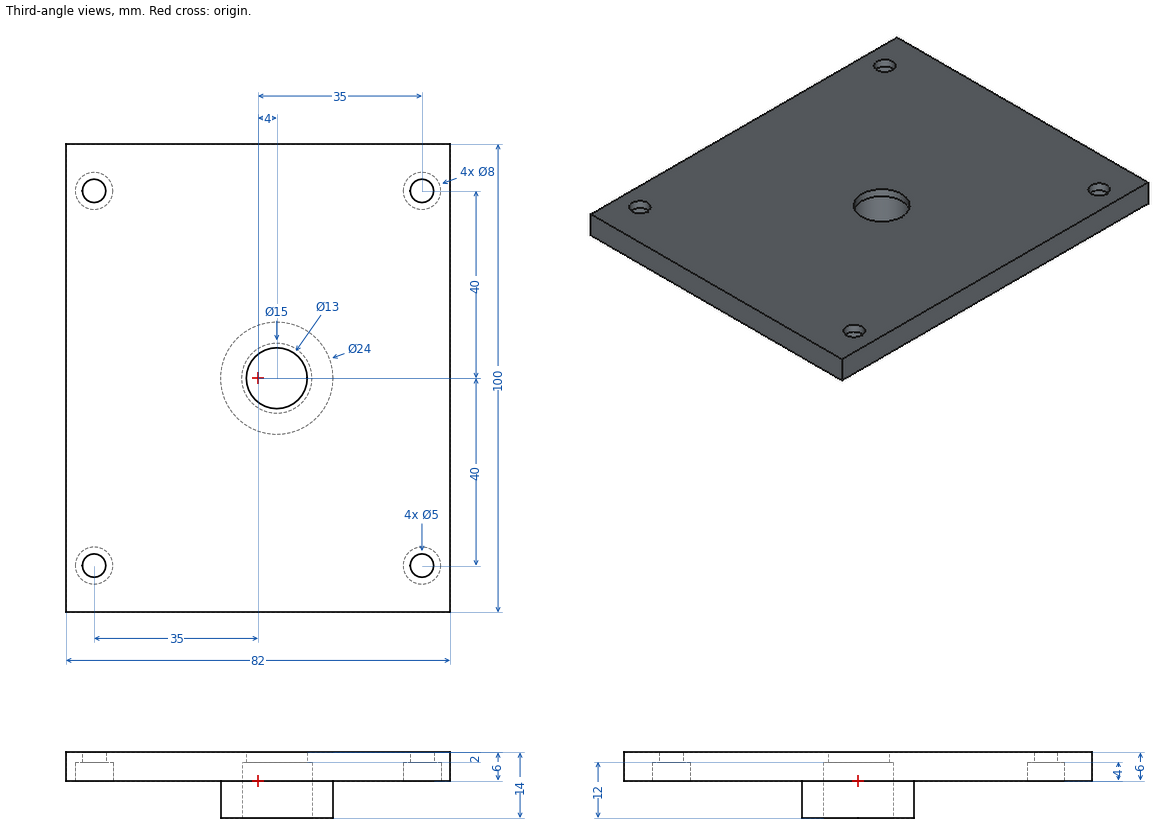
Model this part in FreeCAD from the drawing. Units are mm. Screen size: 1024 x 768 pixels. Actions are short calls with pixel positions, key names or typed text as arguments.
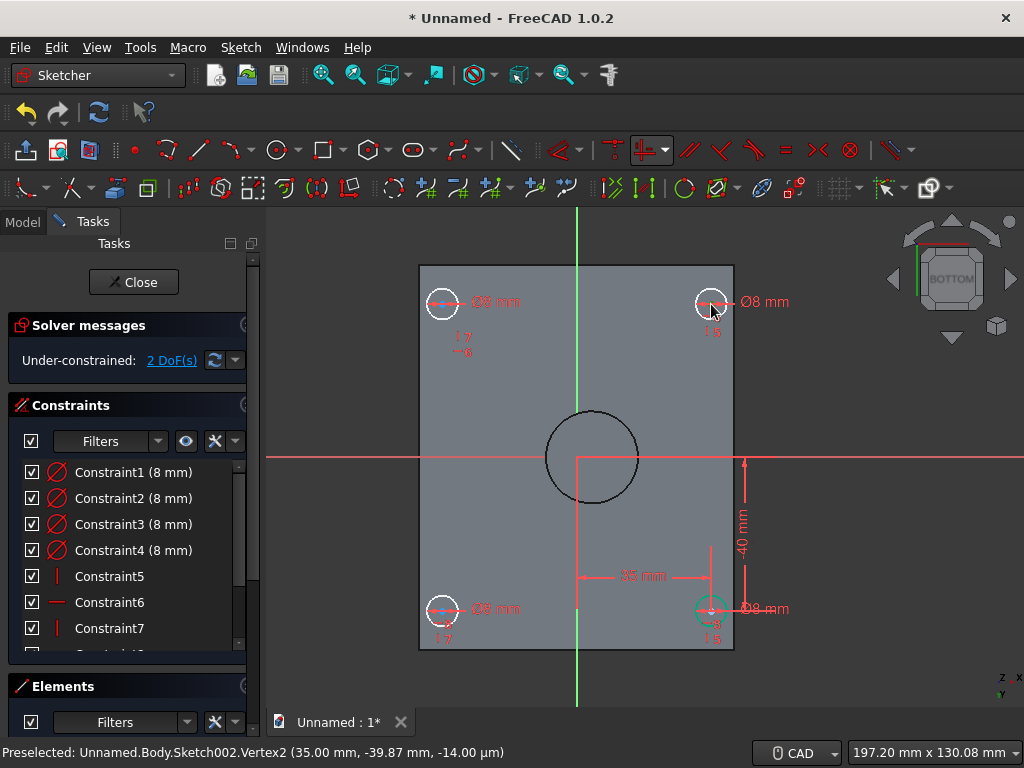
click(582, 150)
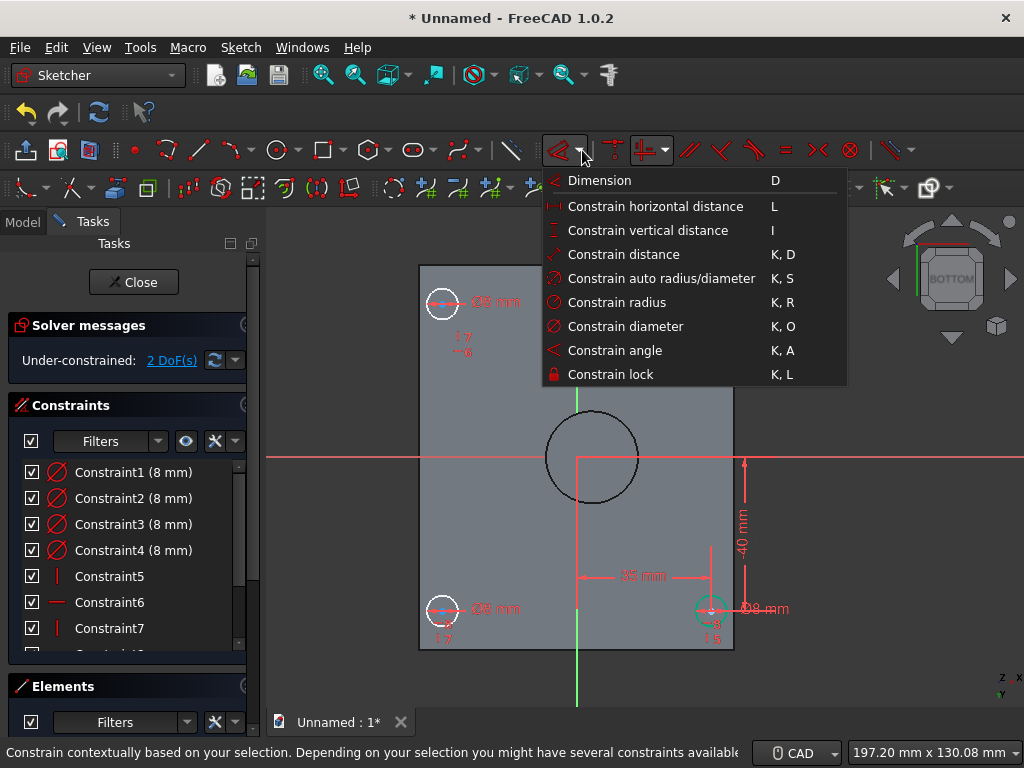
click(695, 230)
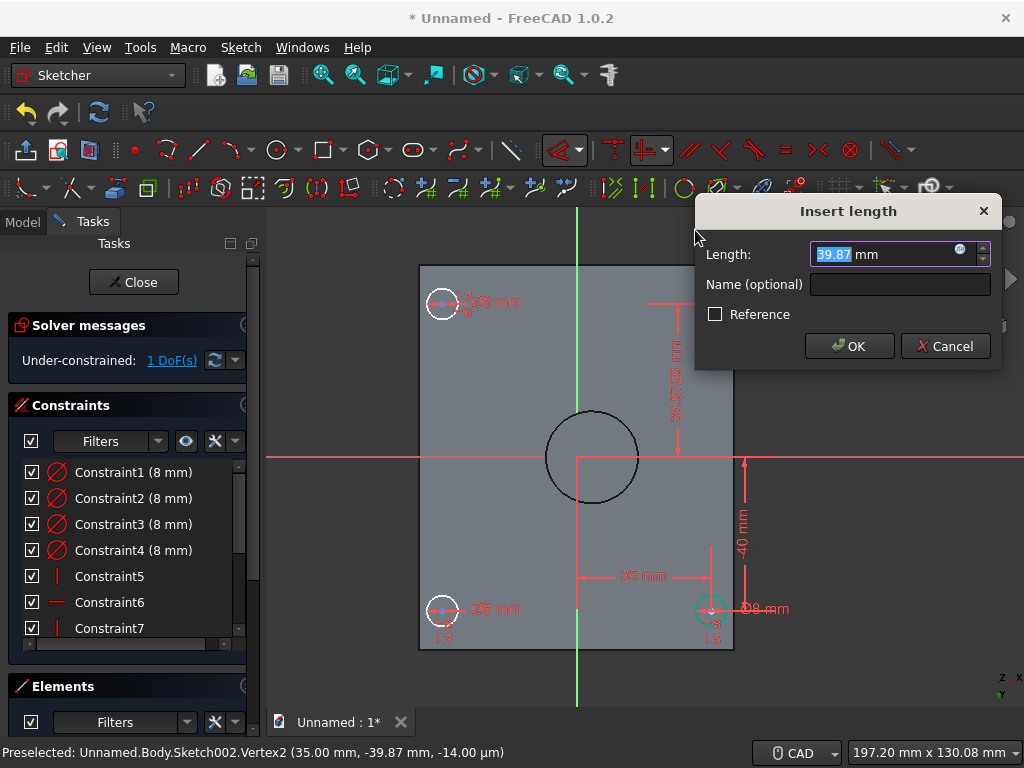
text(40)
key(Return)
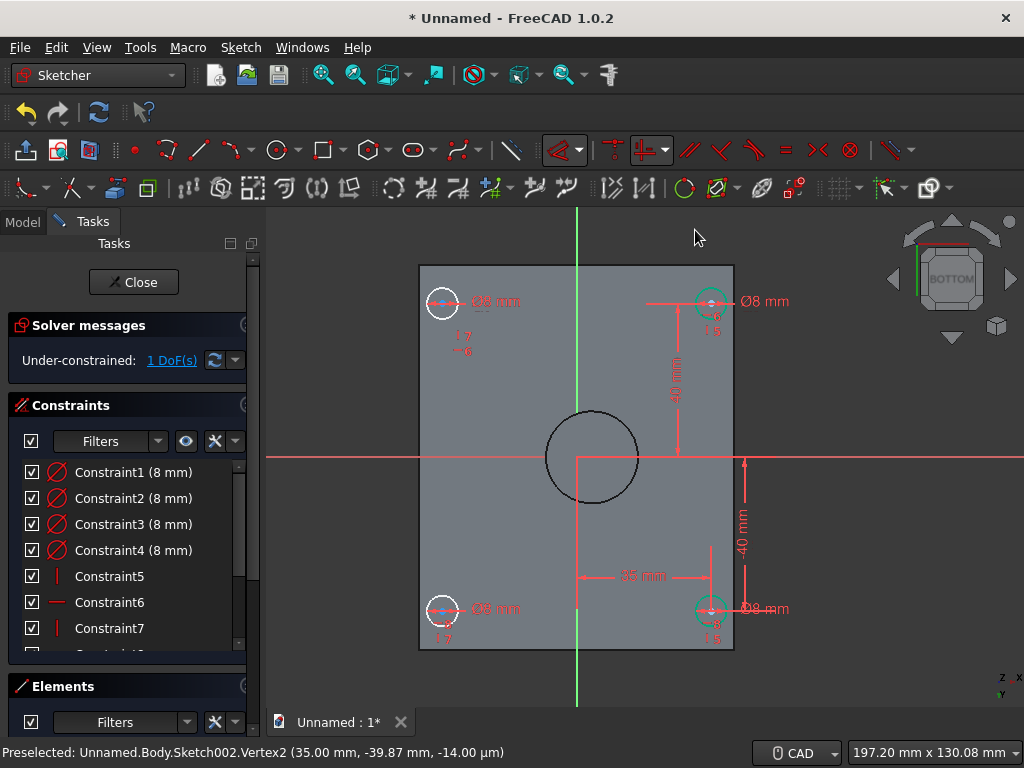
click(442, 304)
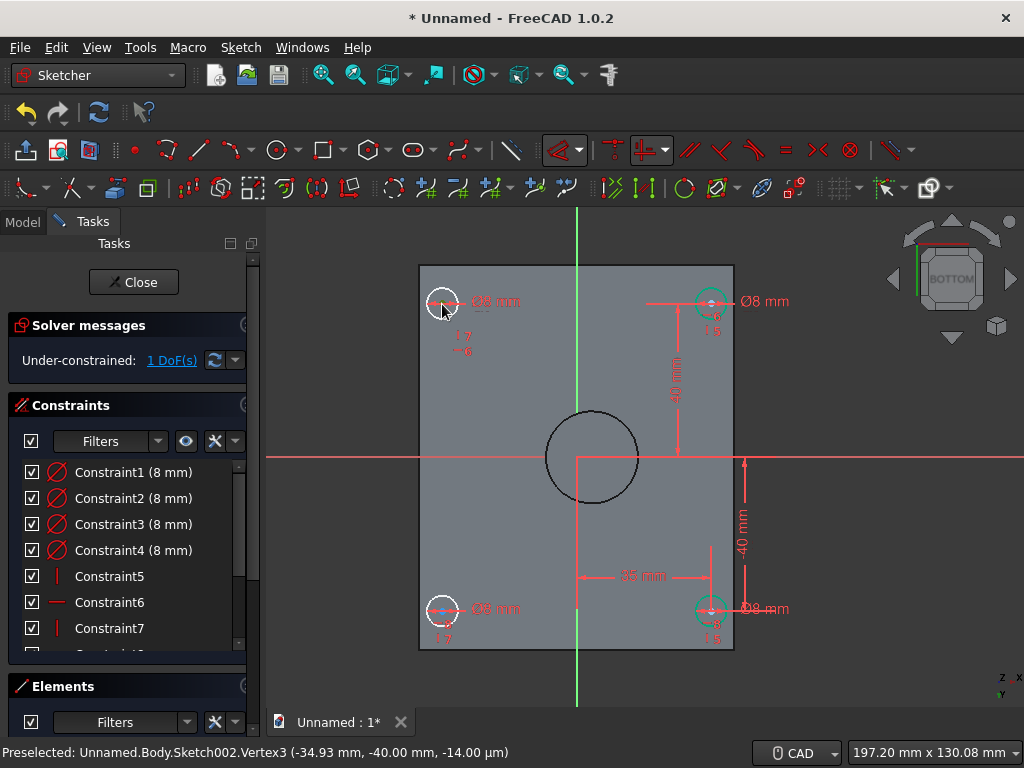
key(l)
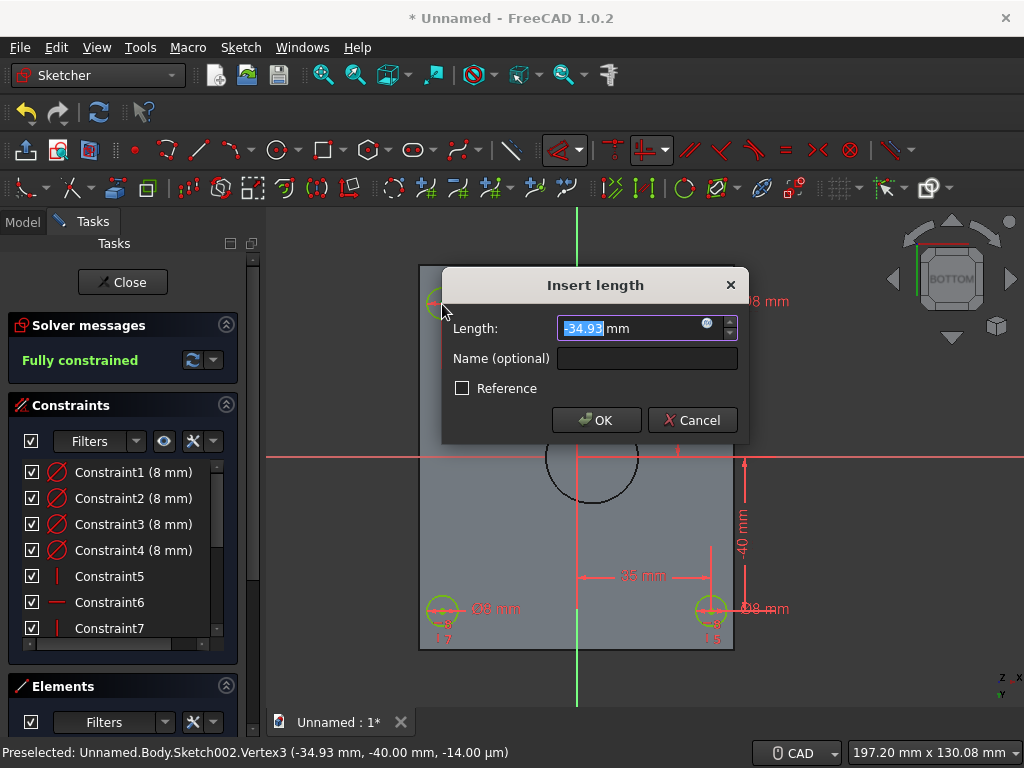
text(-35)
key(Return)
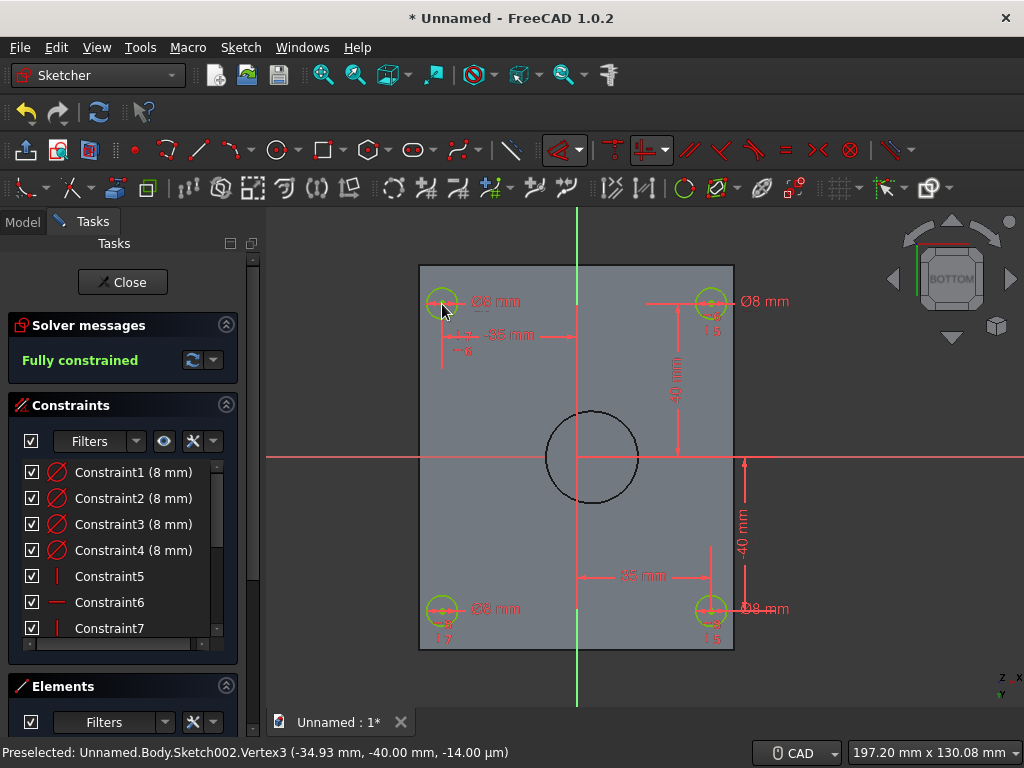
click(123, 282)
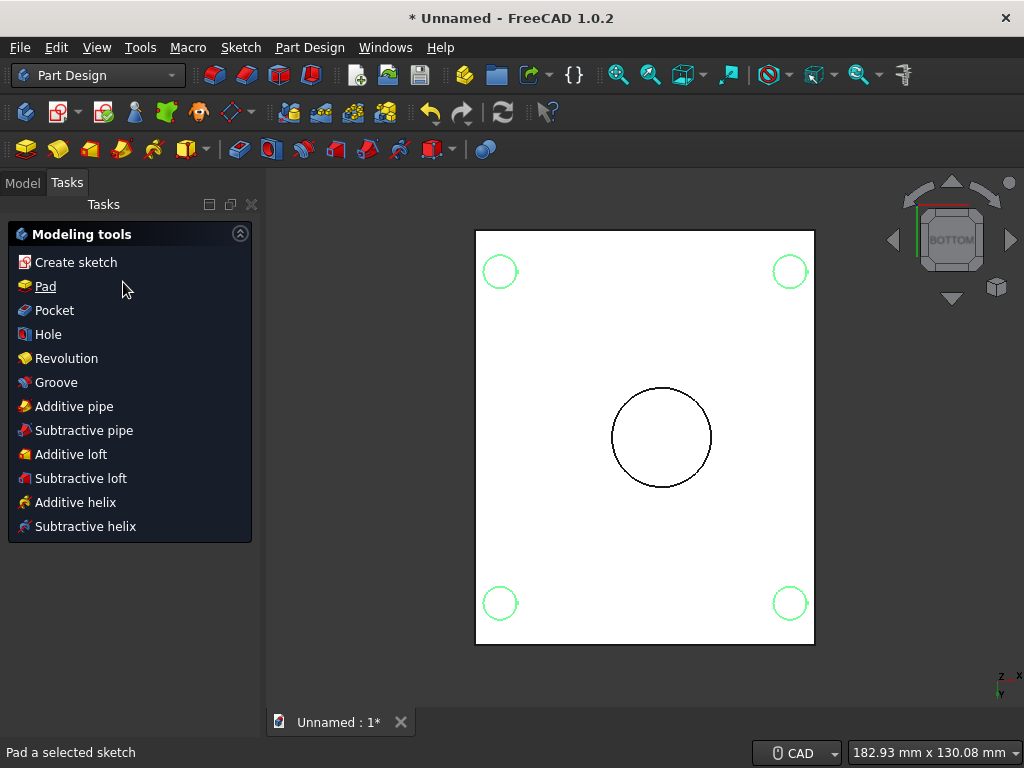
click(240, 150)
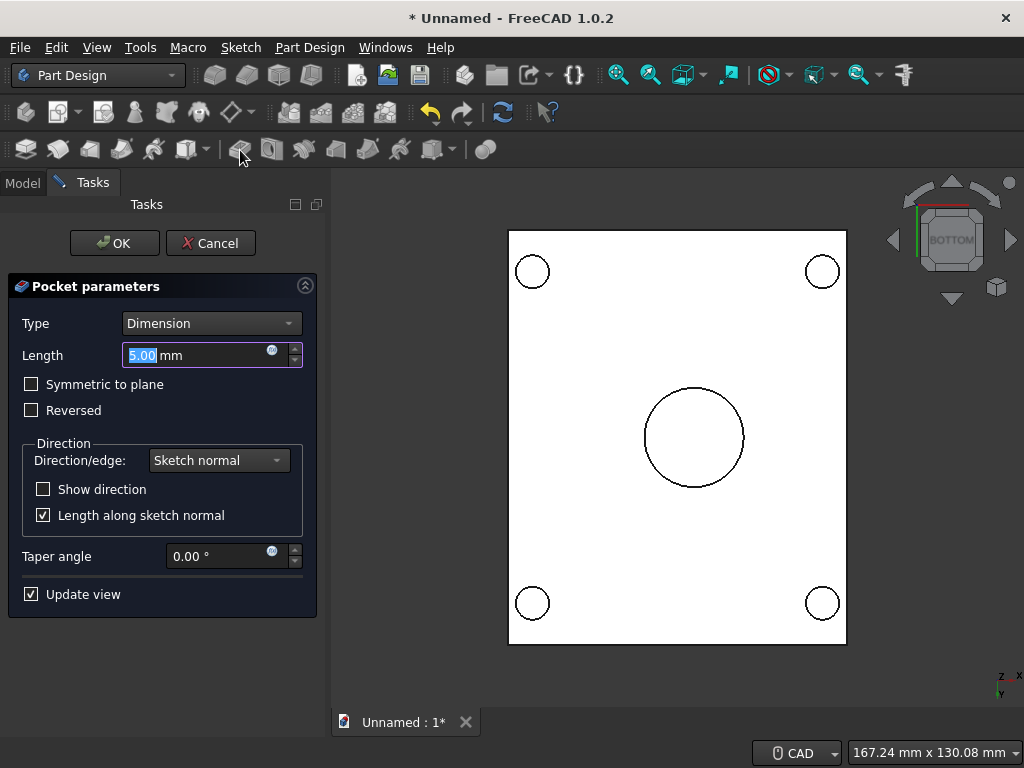
text(4)
key(Tab)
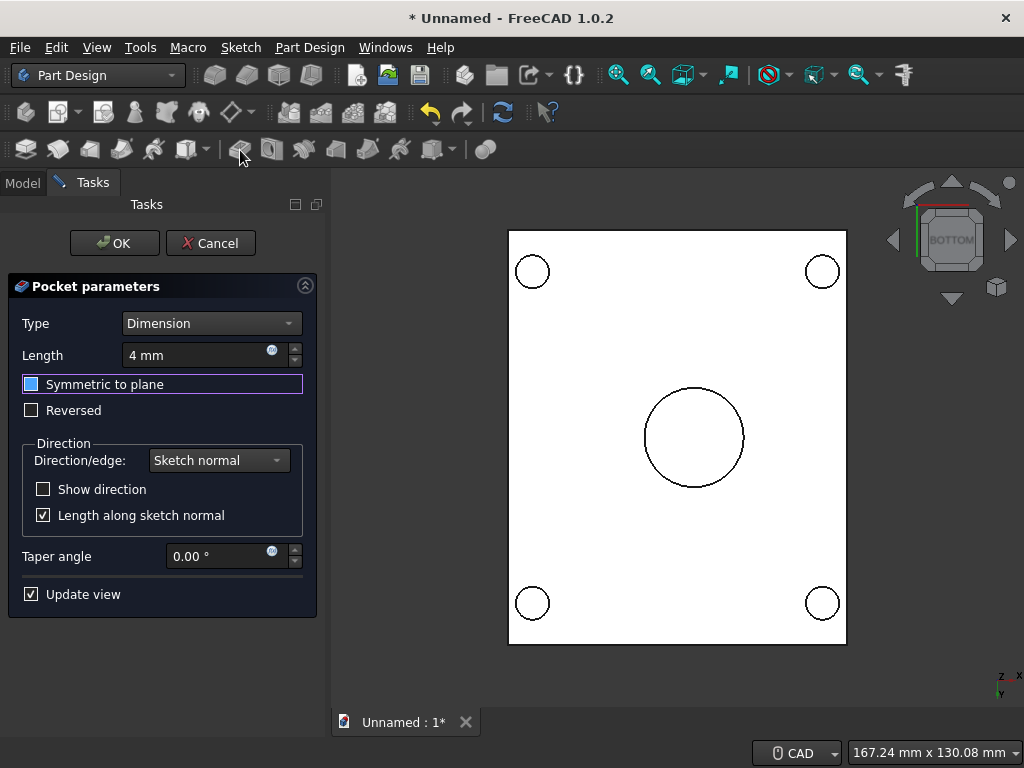
click(115, 243)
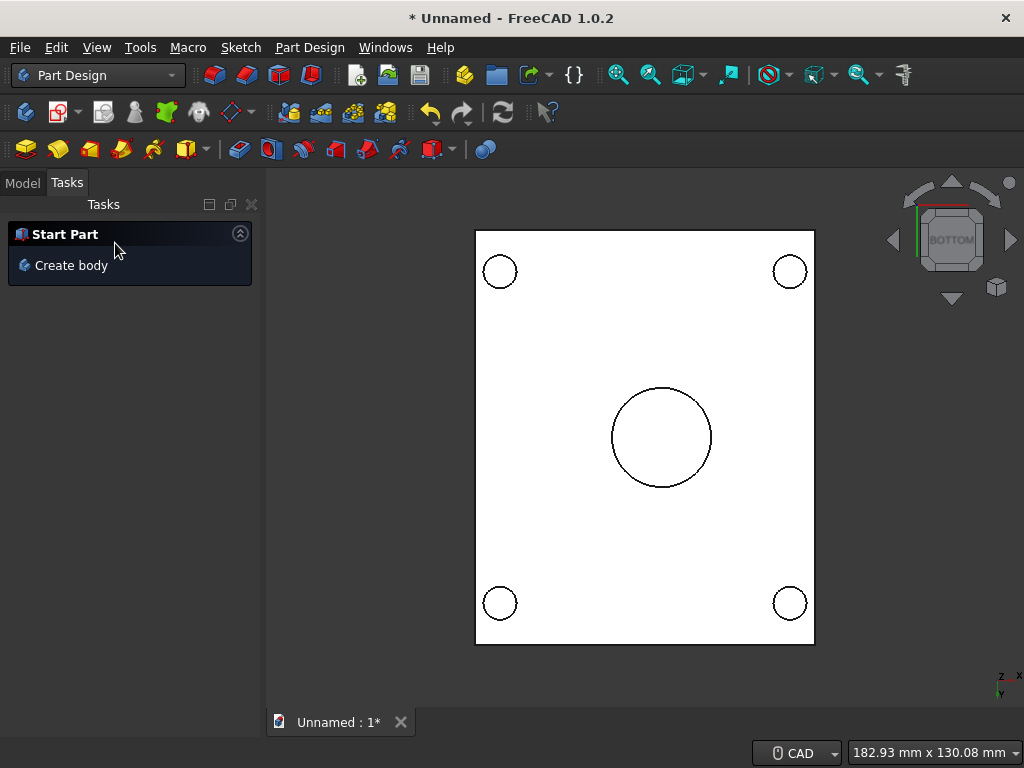
key(0)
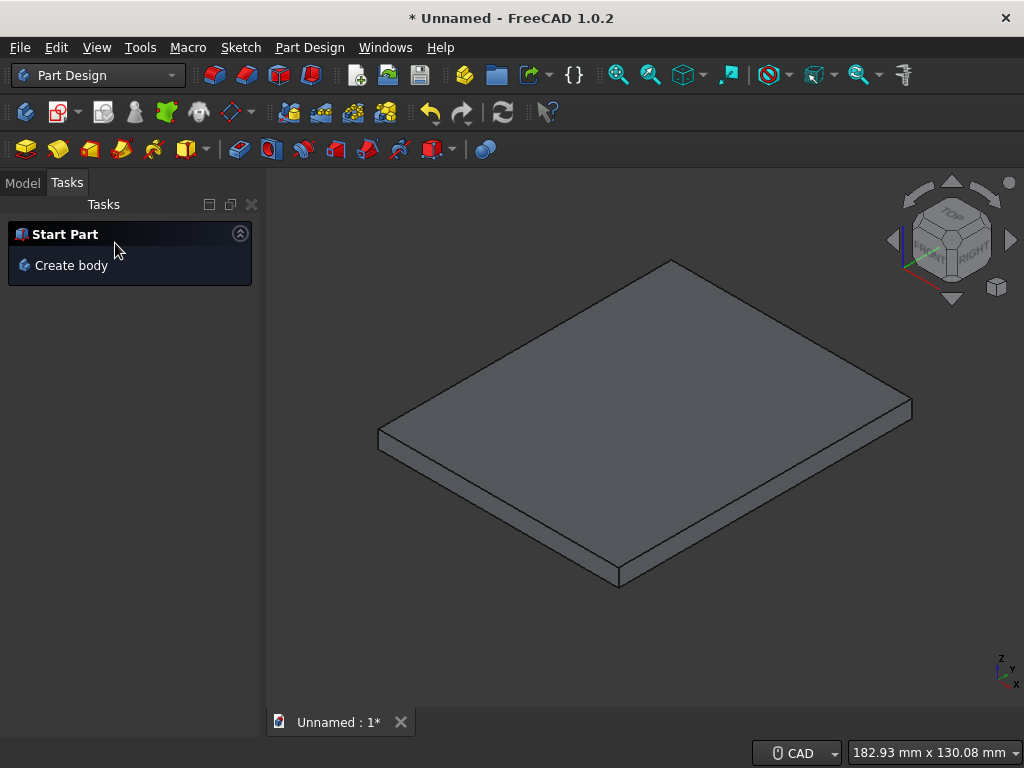
click(645, 413)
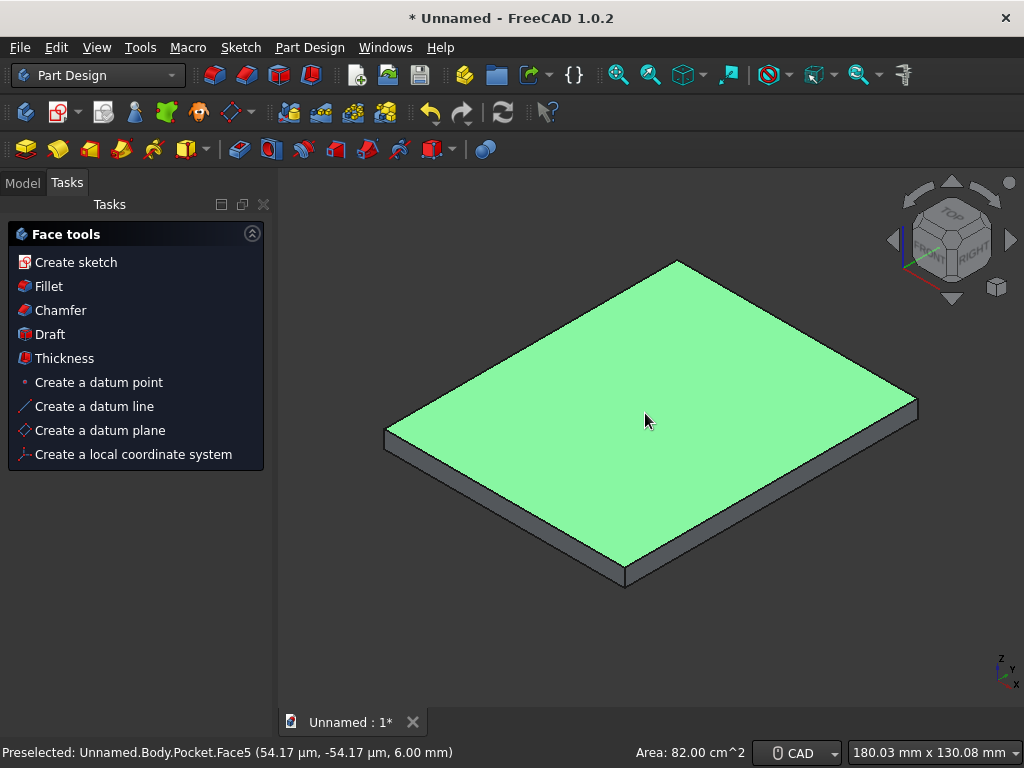
click(58, 112)